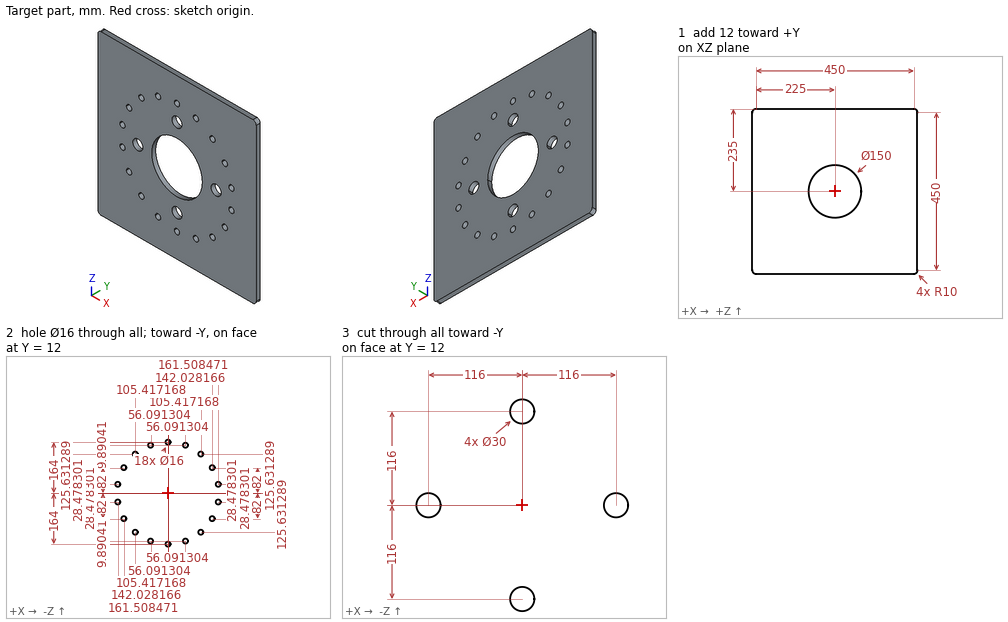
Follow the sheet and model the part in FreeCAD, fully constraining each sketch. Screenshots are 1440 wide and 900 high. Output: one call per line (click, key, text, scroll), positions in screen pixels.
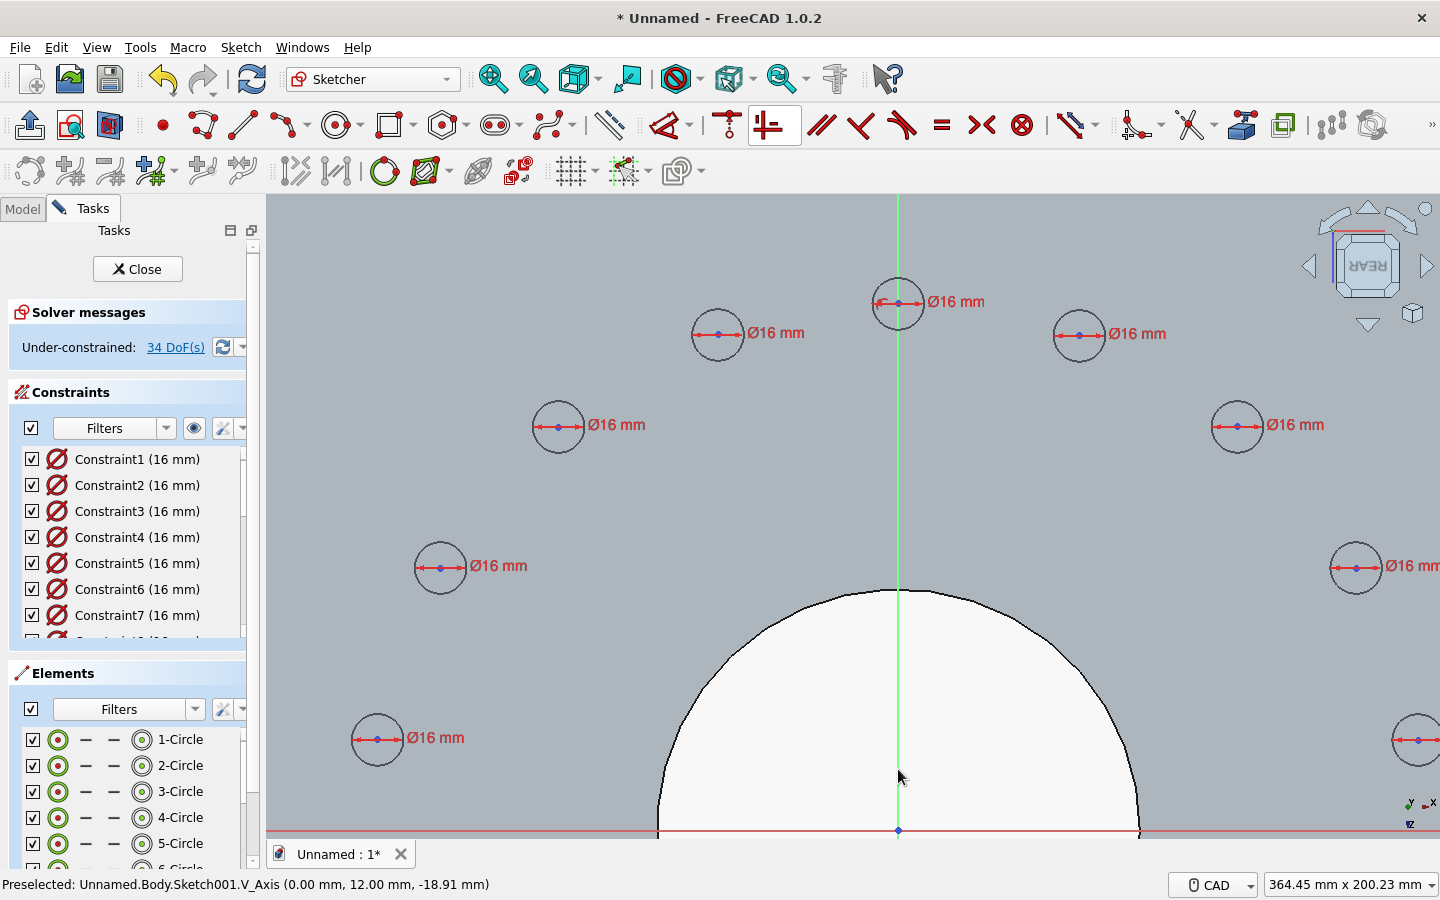
scroll(718, 334, down, 5)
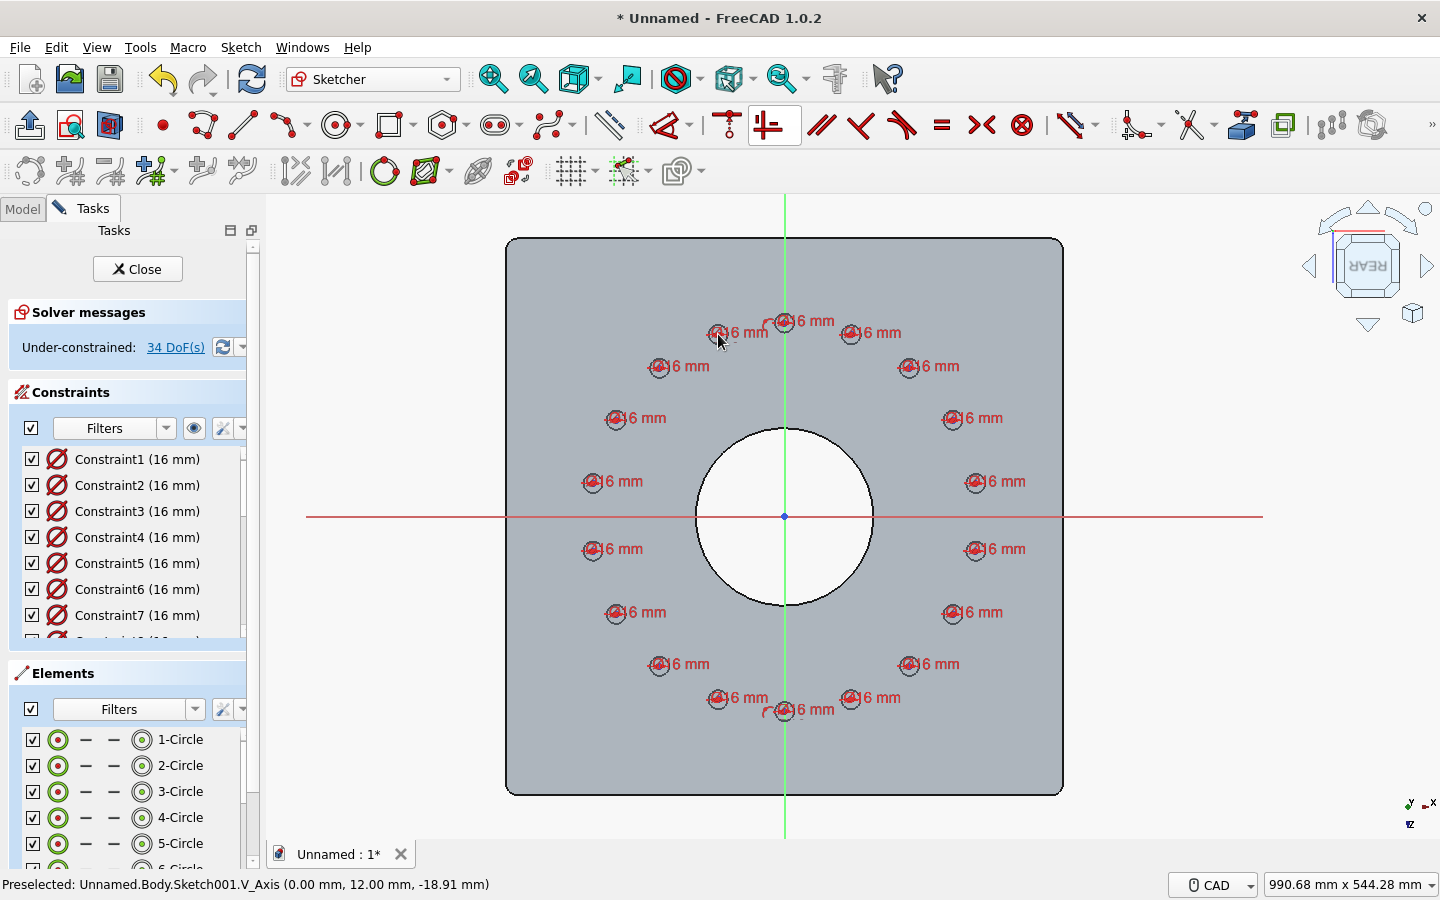
click(976, 483)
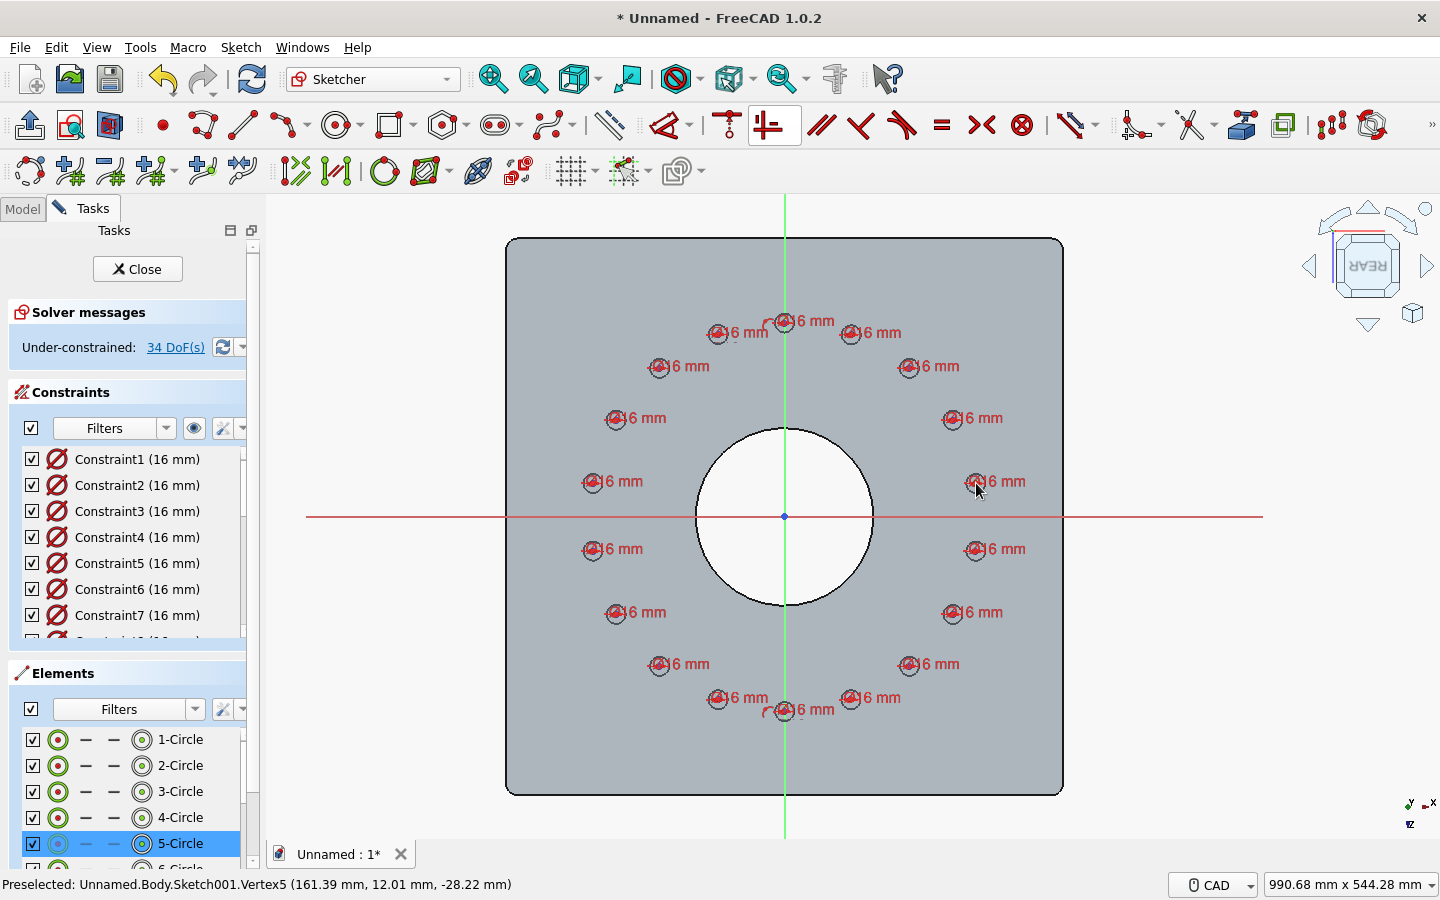
click(976, 551)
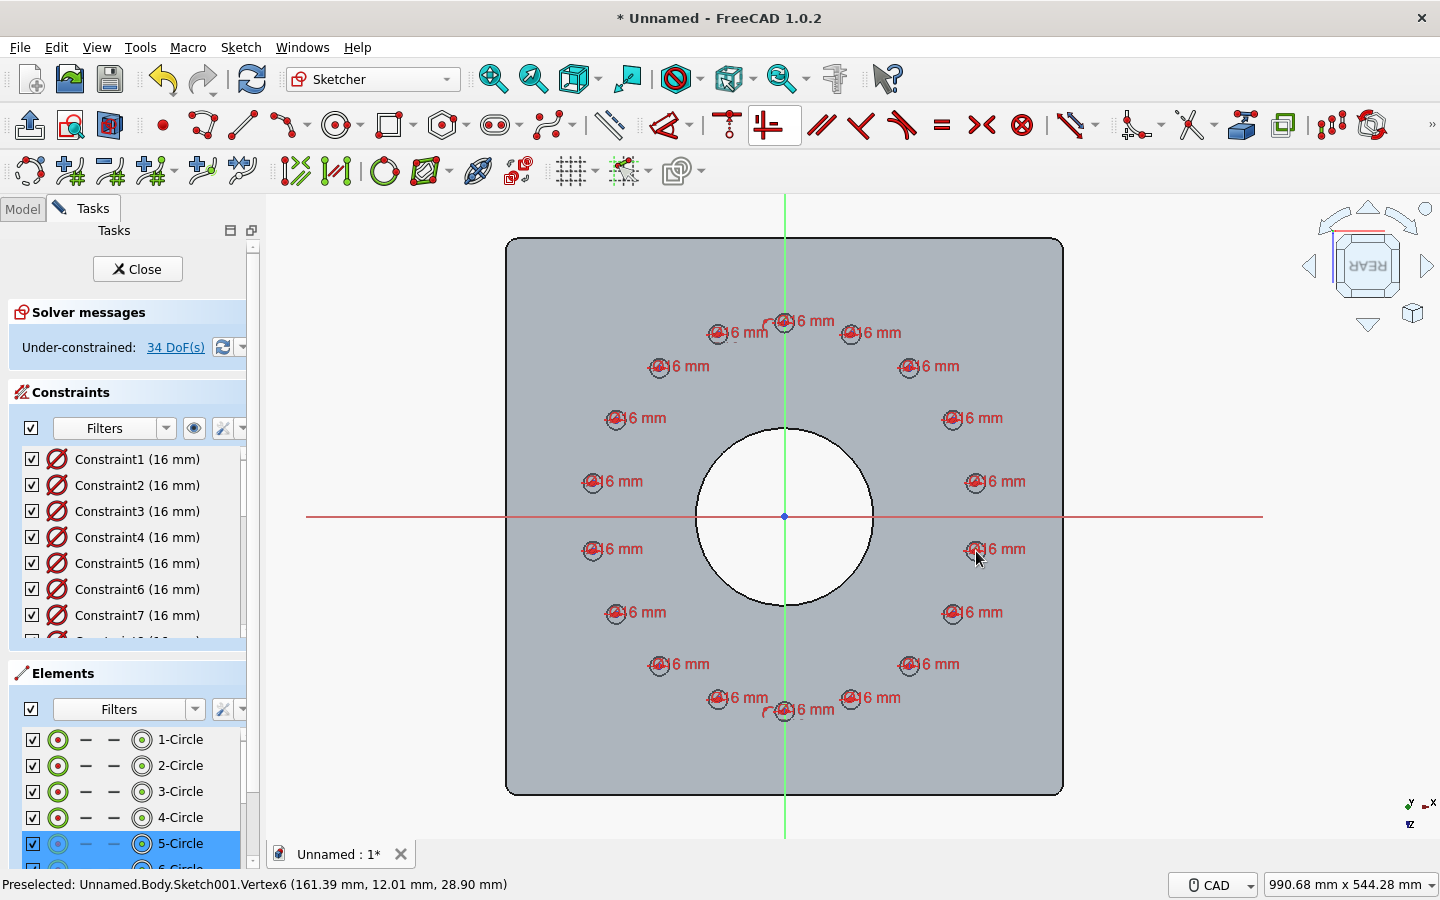
key(v)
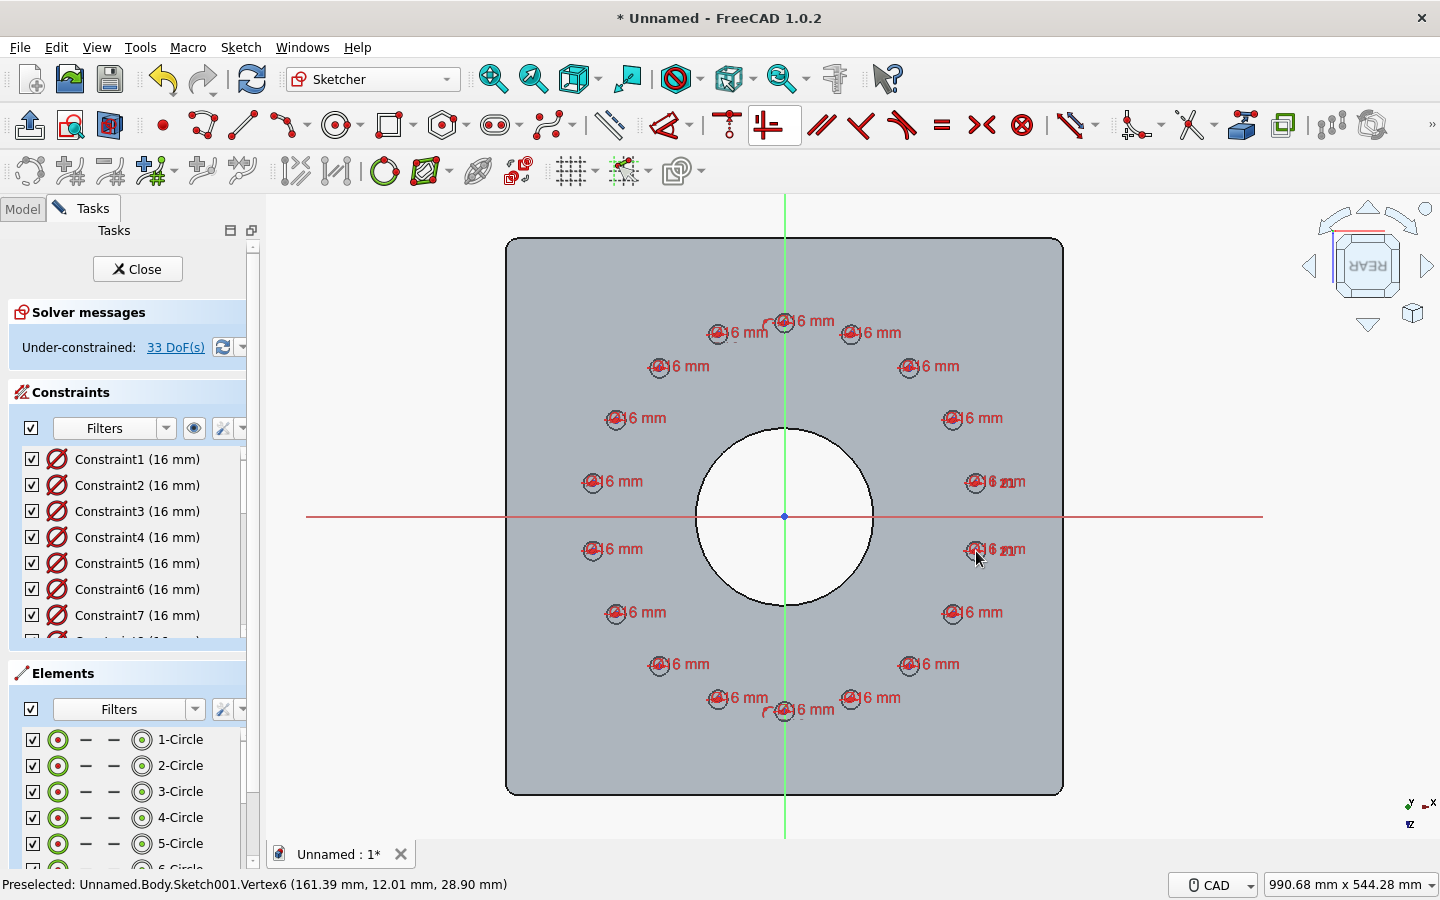
click(953, 420)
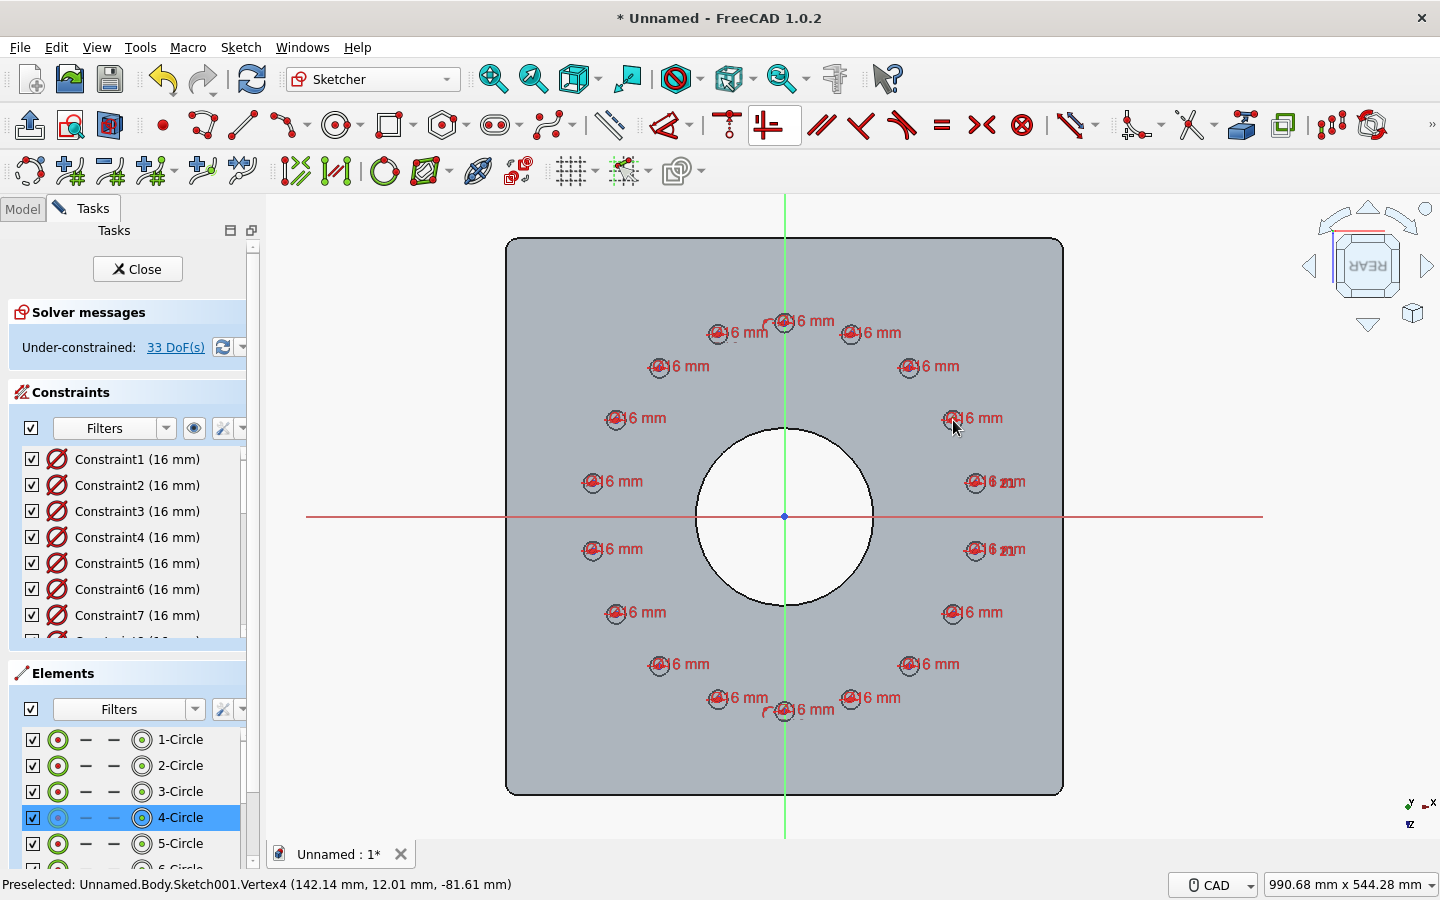
click(953, 614)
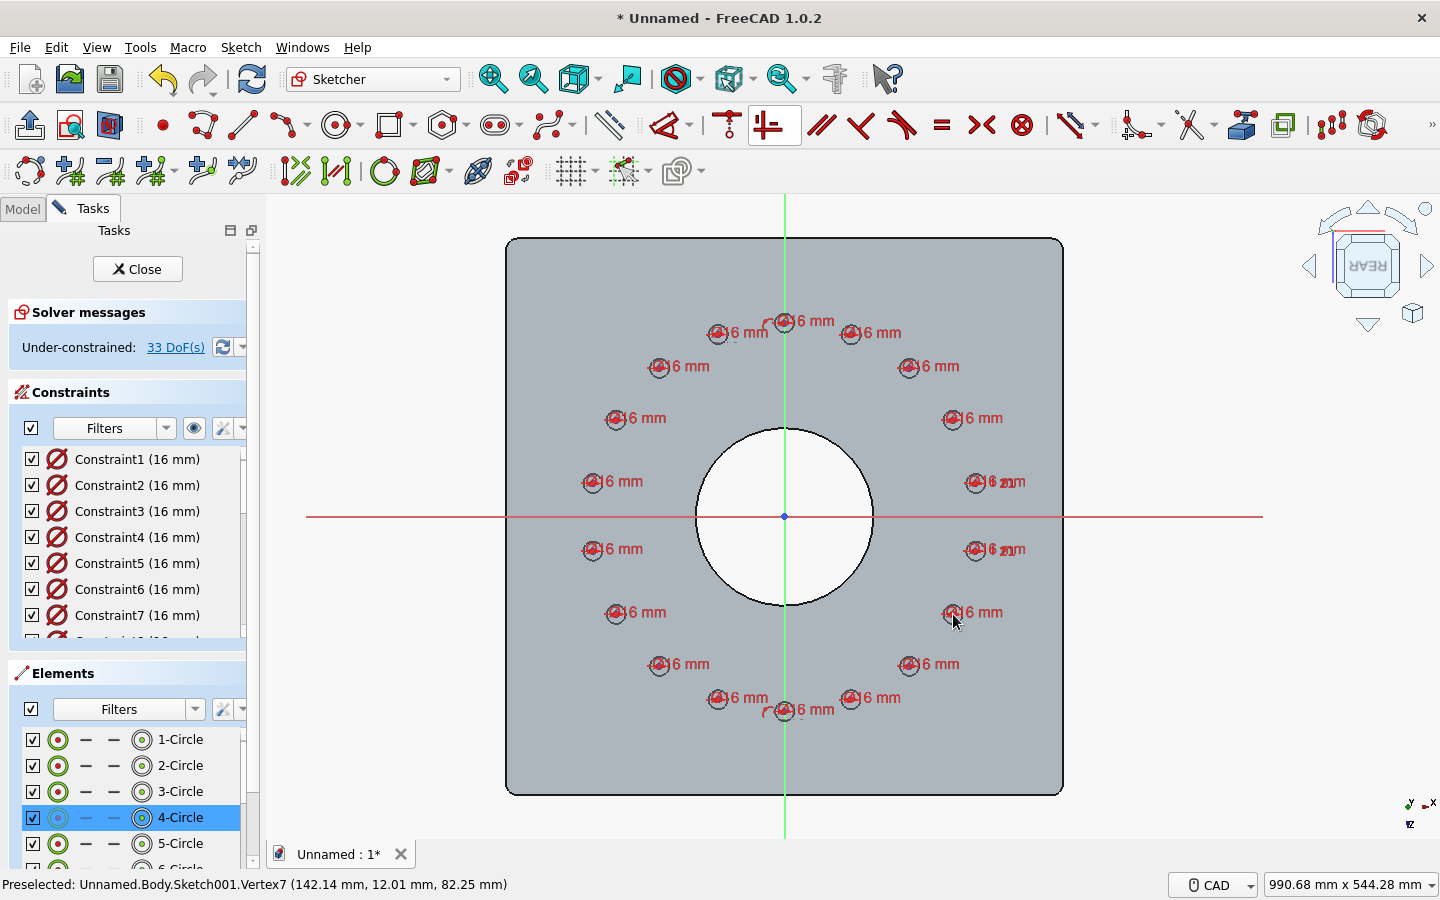
click(796, 126)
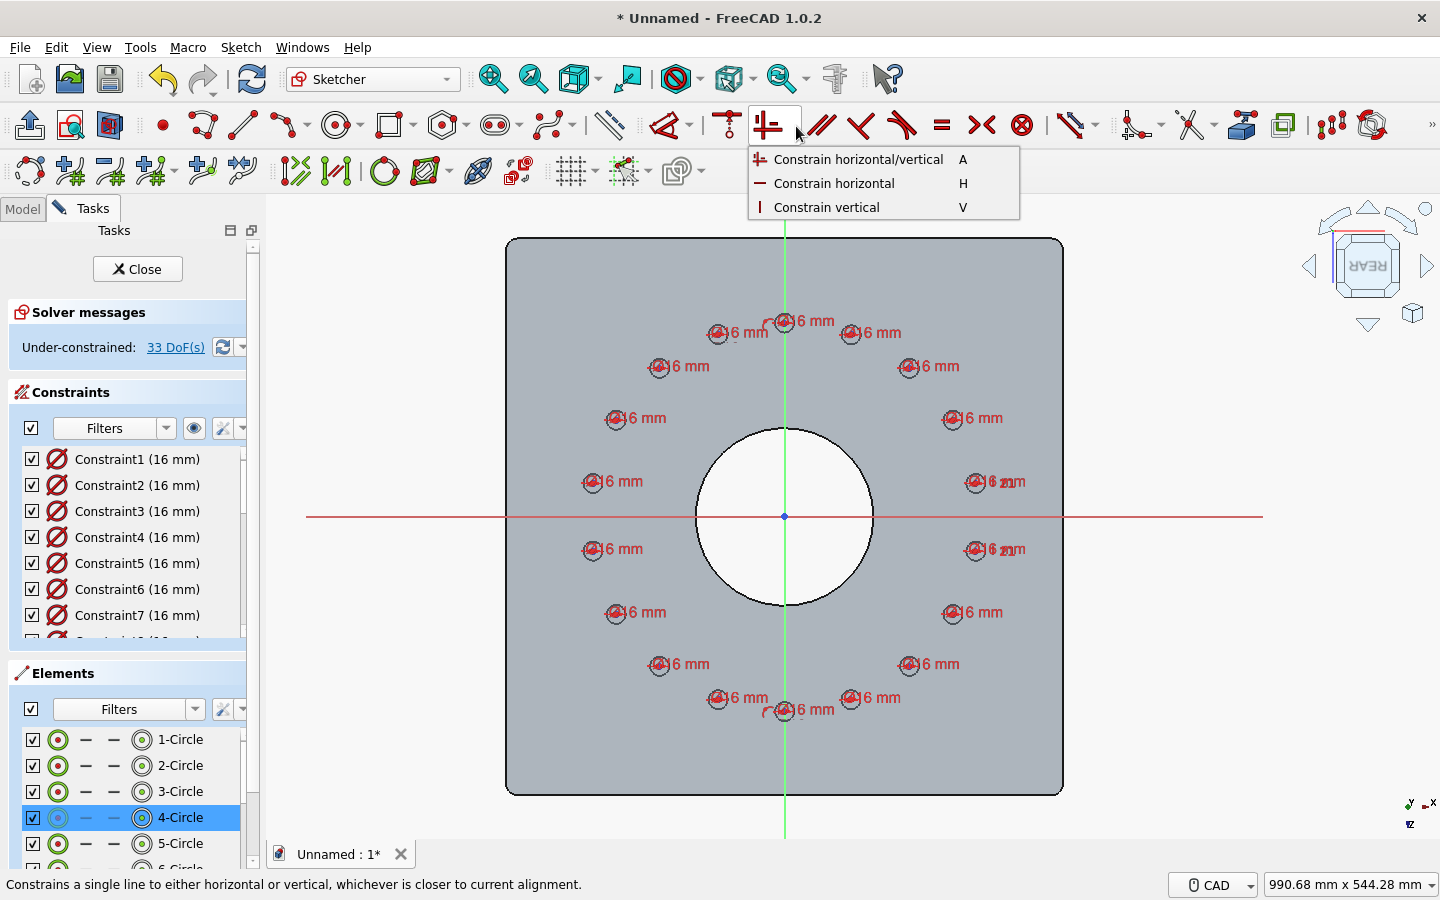
click(884, 207)